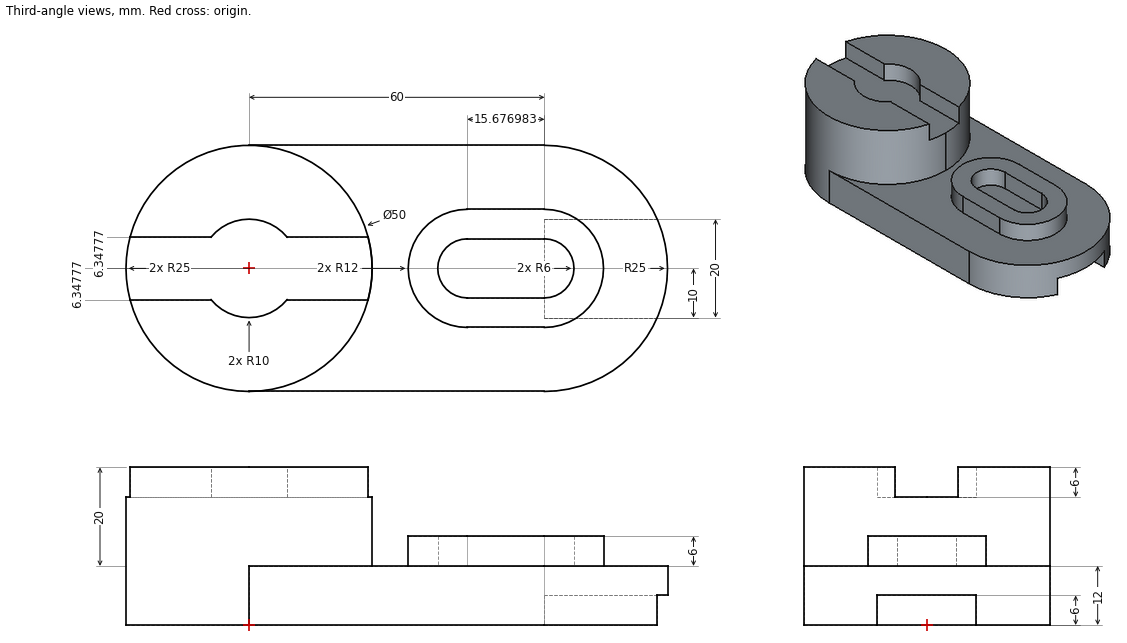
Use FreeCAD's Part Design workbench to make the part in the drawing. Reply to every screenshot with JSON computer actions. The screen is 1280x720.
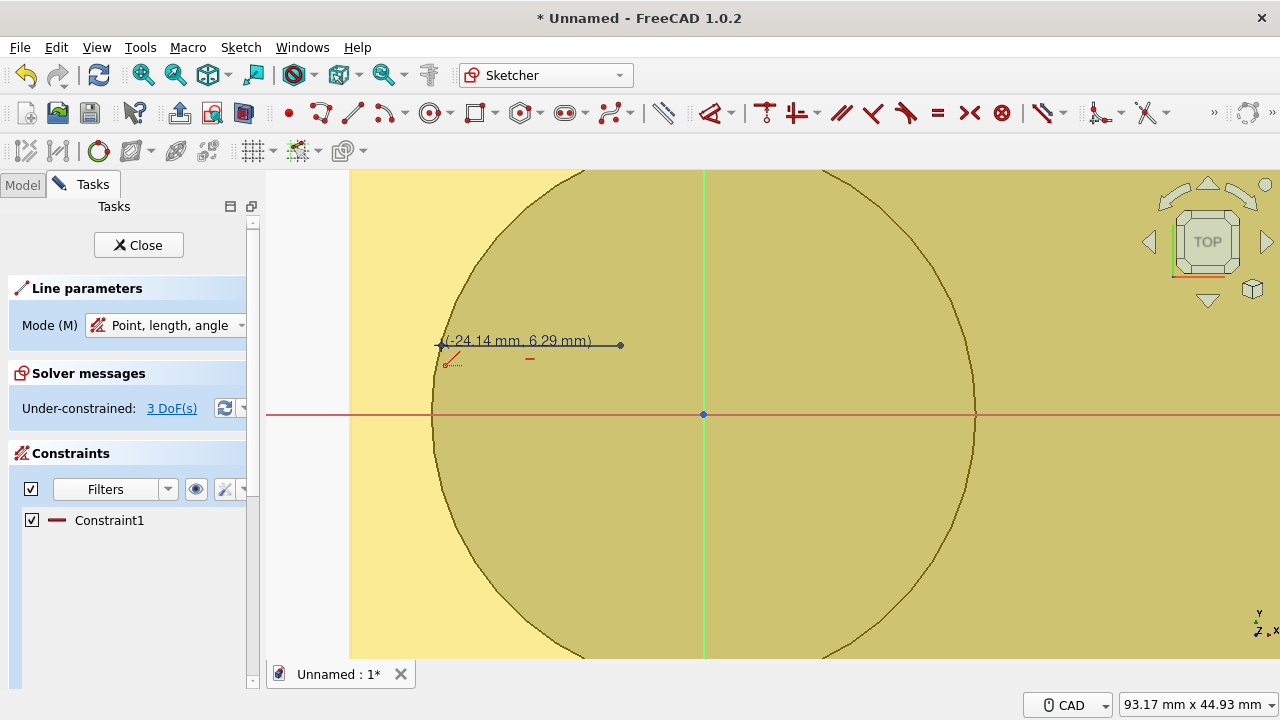
{"action": "left_click", "coordinate": [441, 484]}
{"action": "left_click", "coordinate": [620, 484]}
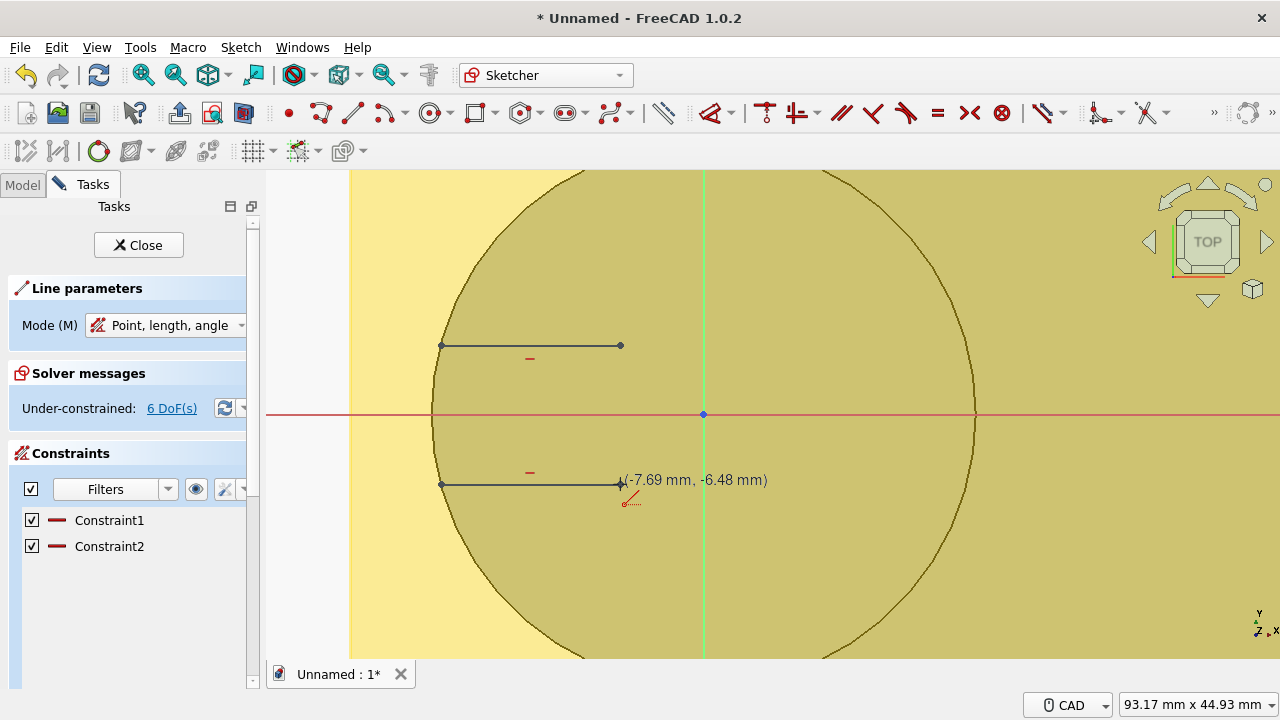
{"action": "left_click", "coordinate": [788, 484]}
{"action": "left_click", "coordinate": [967, 484]}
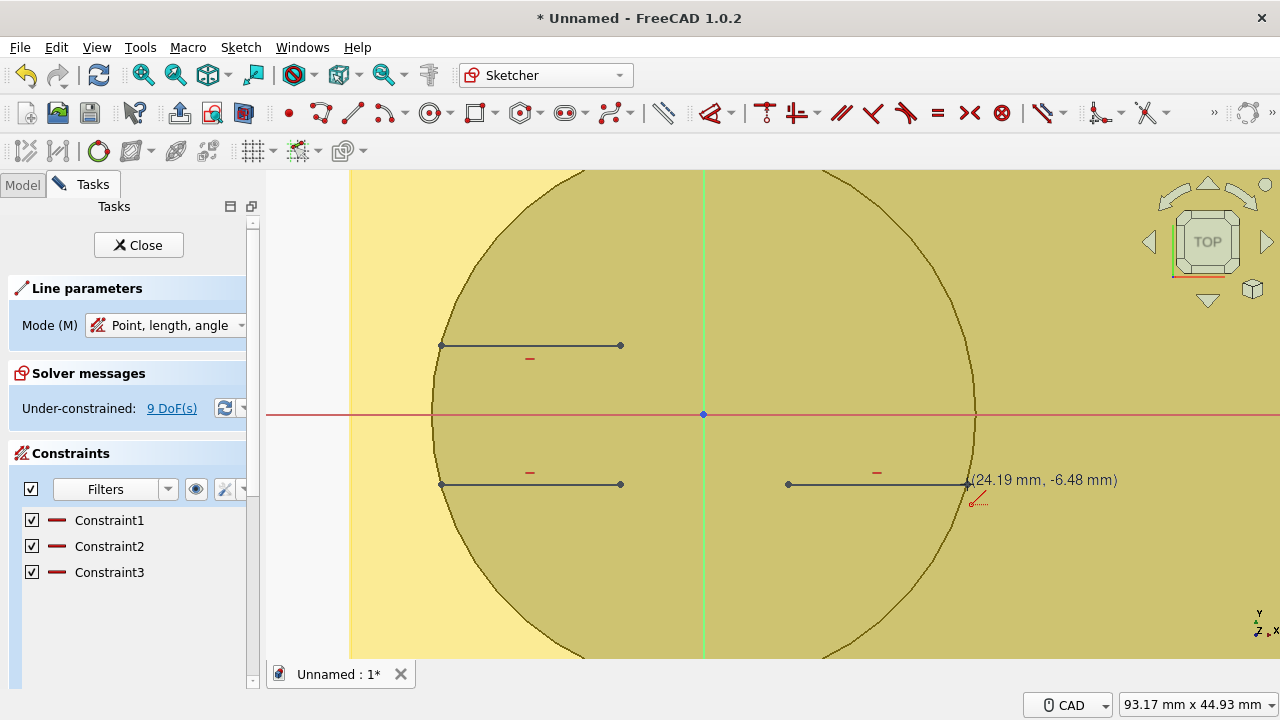
{"action": "left_click", "coordinate": [967, 345]}
{"action": "left_click", "coordinate": [788, 345]}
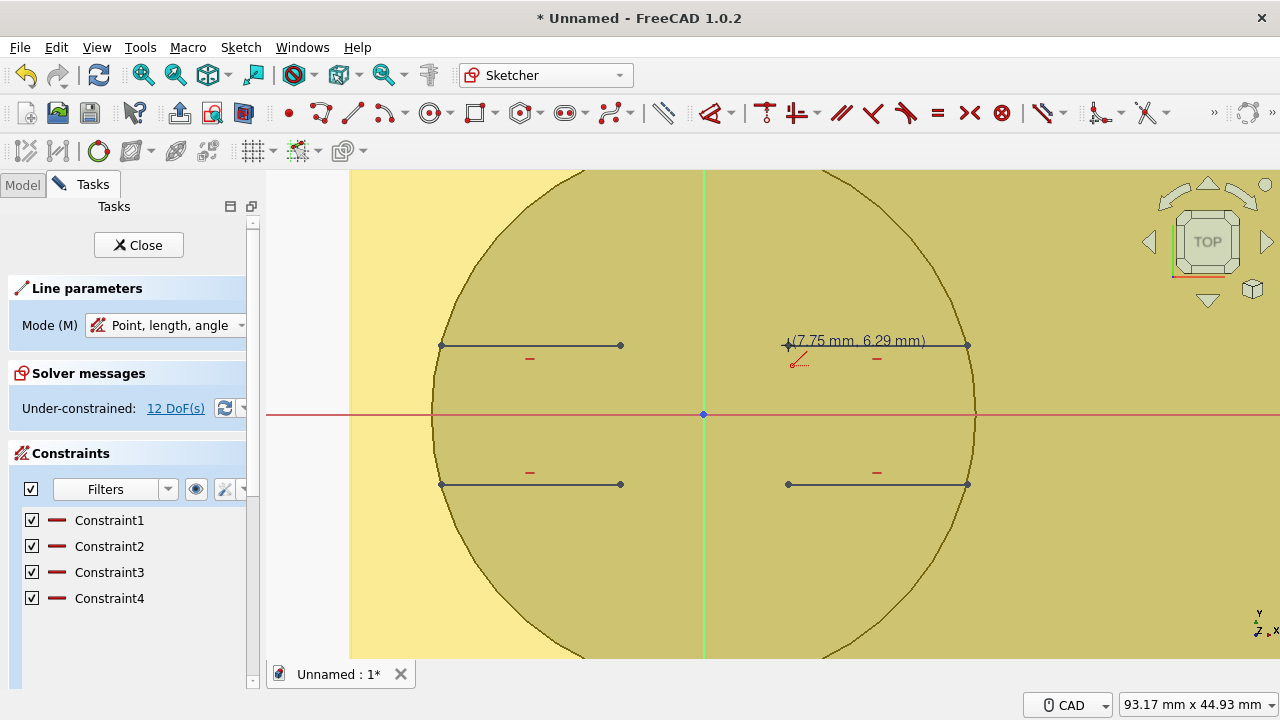
{"action": "key", "text": "g 3 a"}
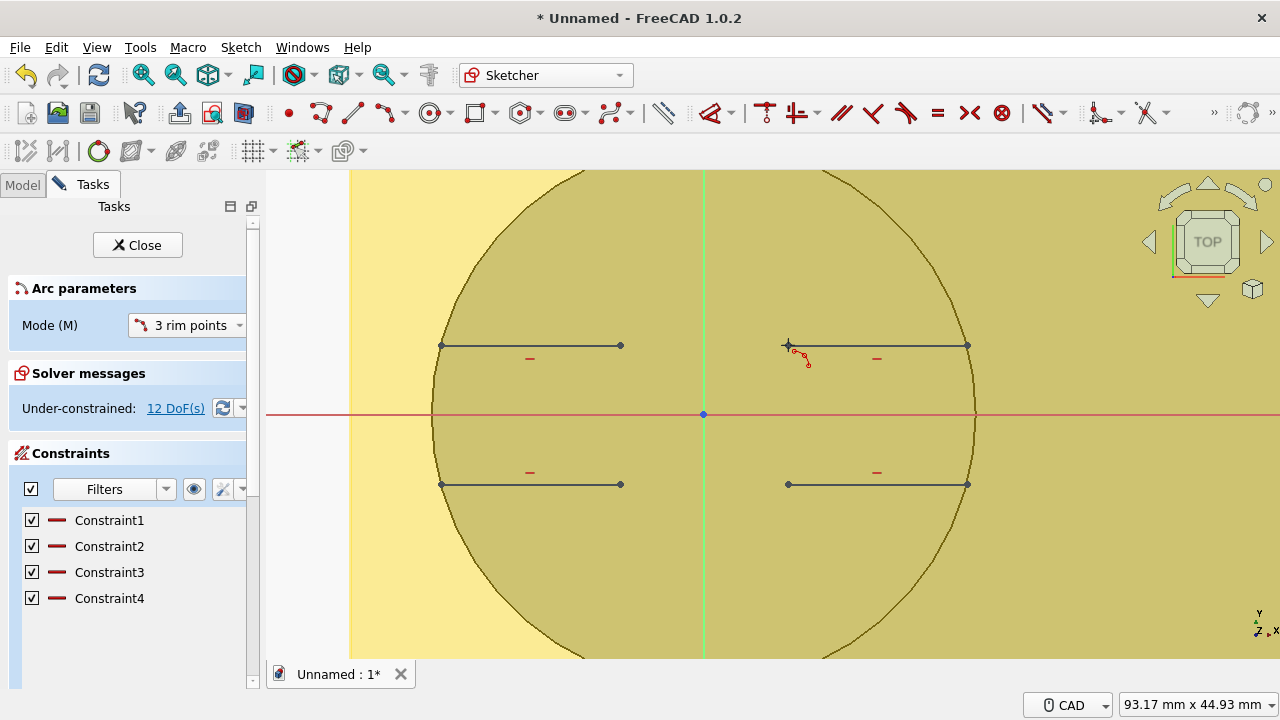
{"action": "left_click", "coordinate": [441, 346]}
{"action": "left_click", "coordinate": [441, 485]}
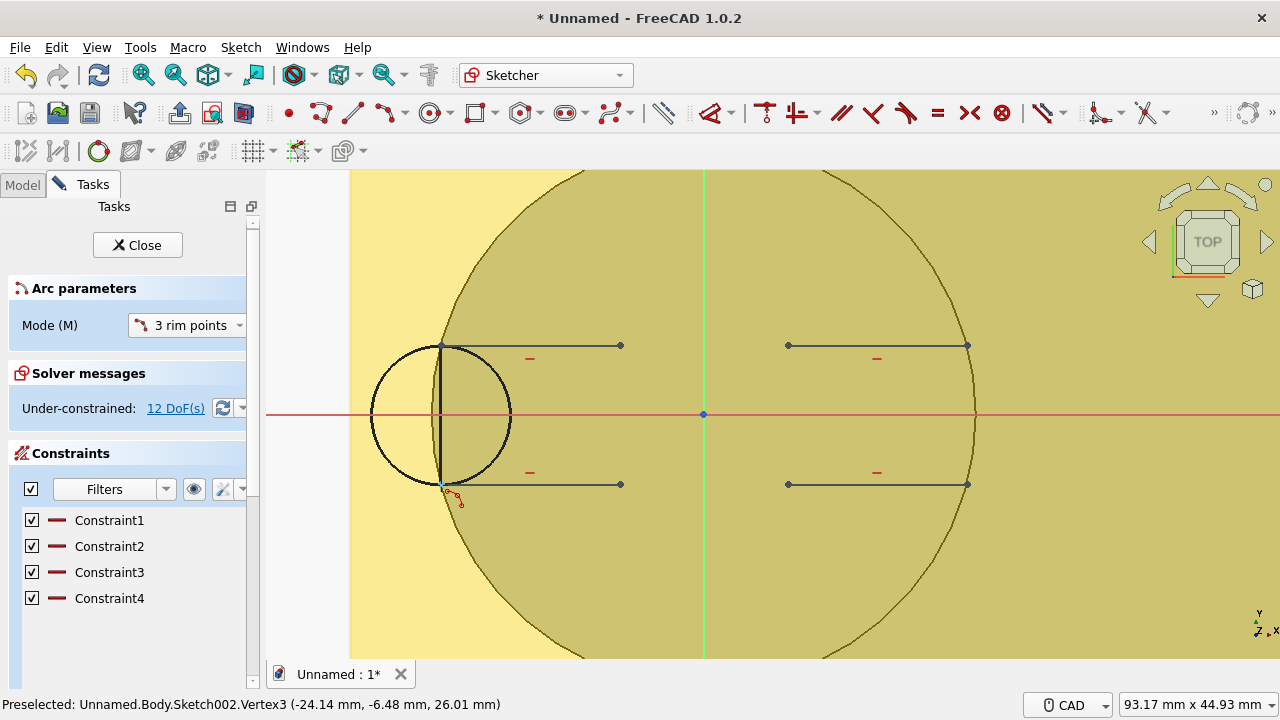
{"action": "scroll", "coordinate": [432, 401], "scroll_direction": "up", "scroll_amount": 4}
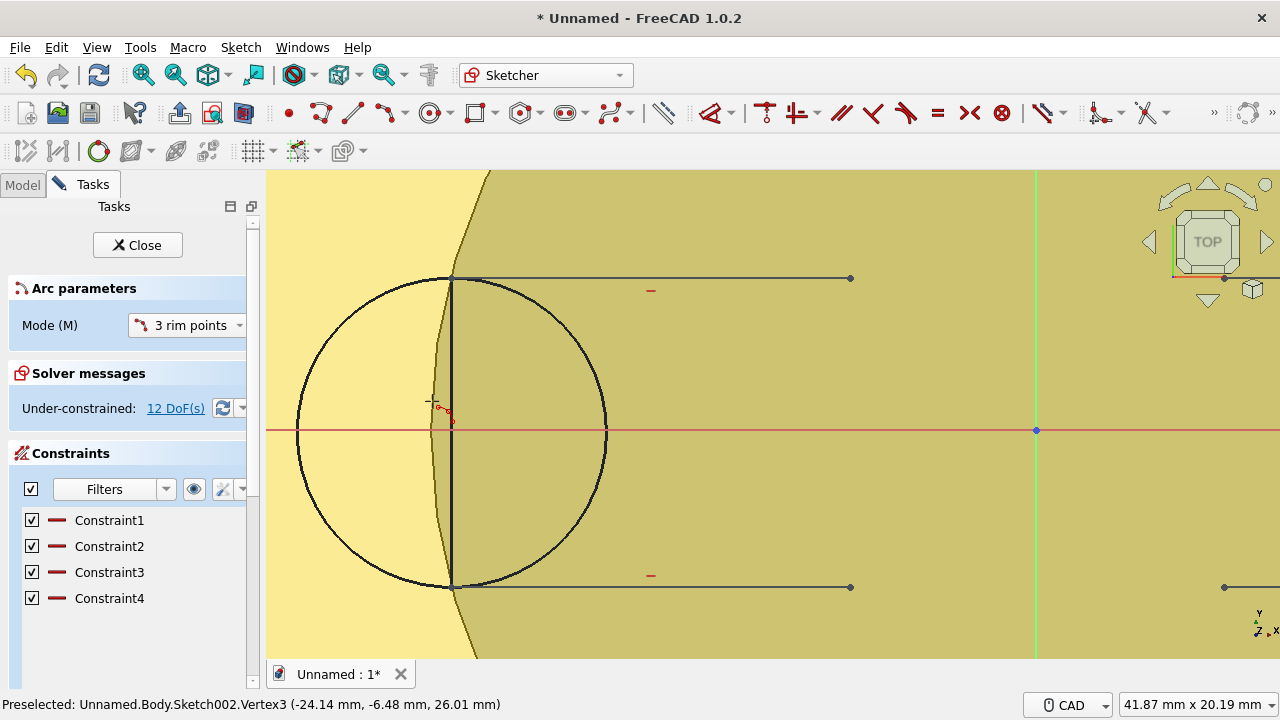
{"action": "left_click", "coordinate": [432, 399]}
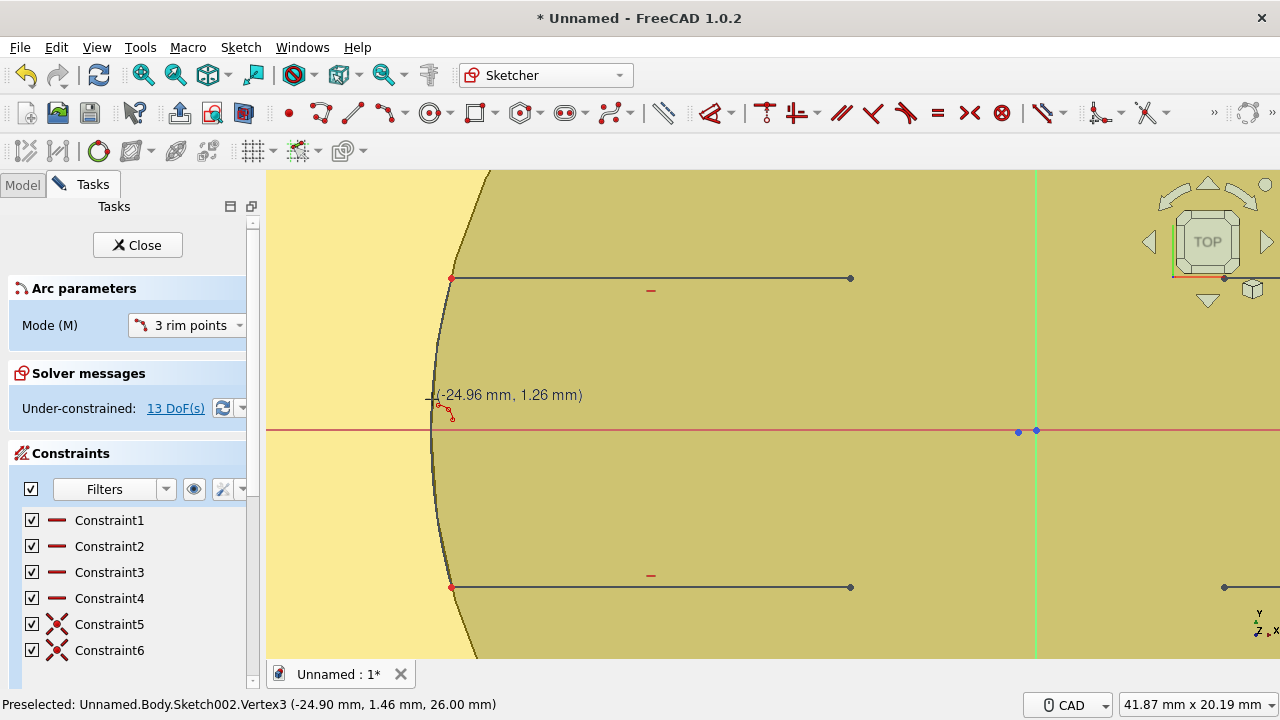
{"action": "left_click", "coordinate": [850, 587]}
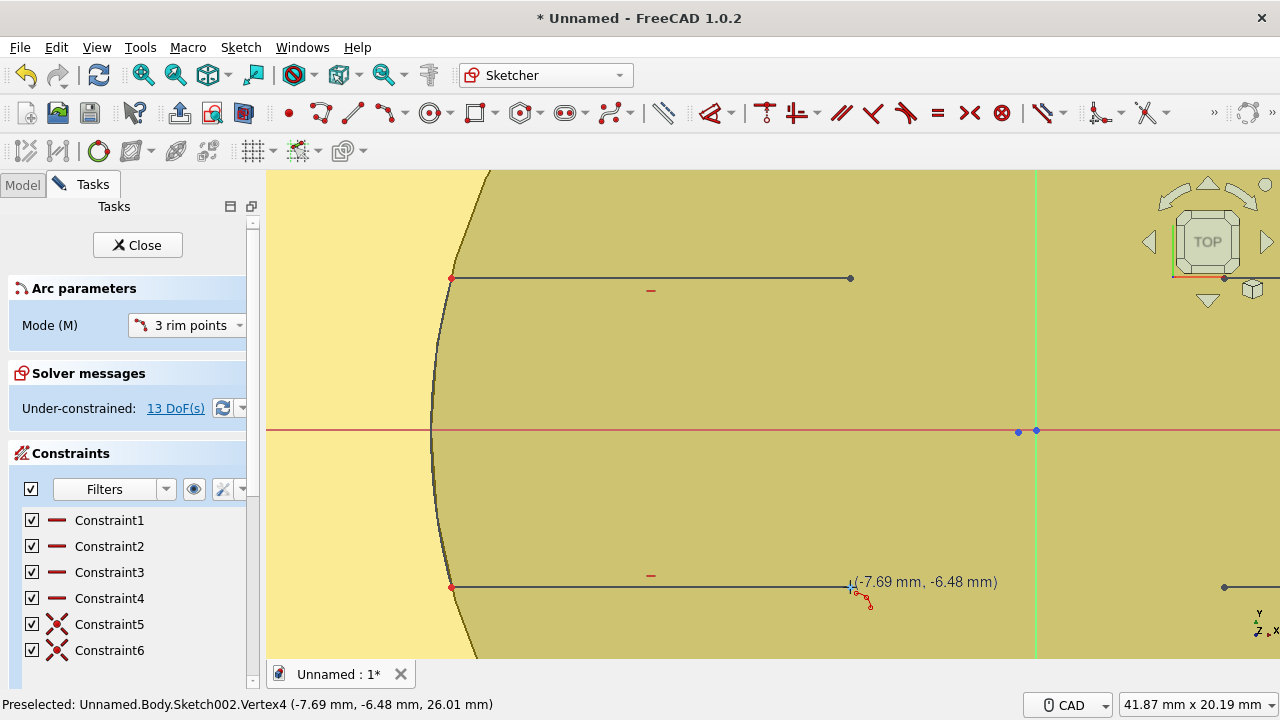
{"action": "scroll", "coordinate": [434, 401], "scroll_direction": "down", "scroll_amount": 4}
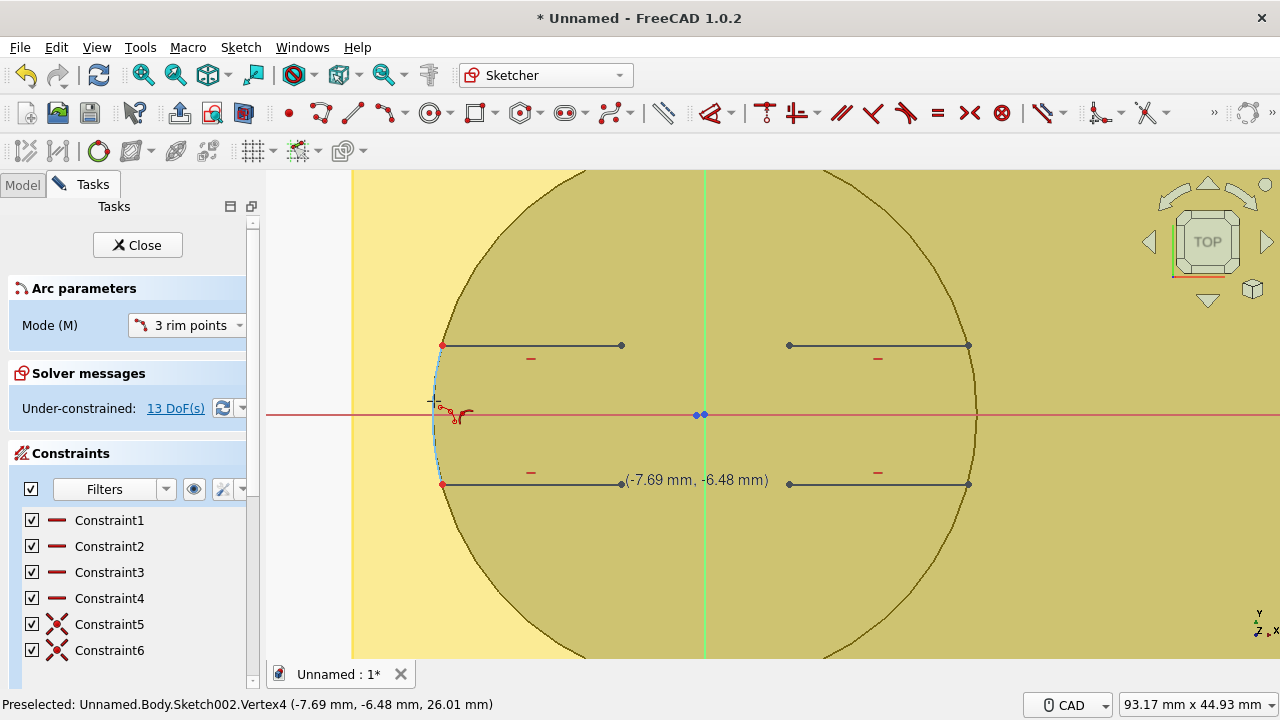
{"action": "left_click", "coordinate": [789, 485]}
{"action": "left_click", "coordinate": [686, 522]}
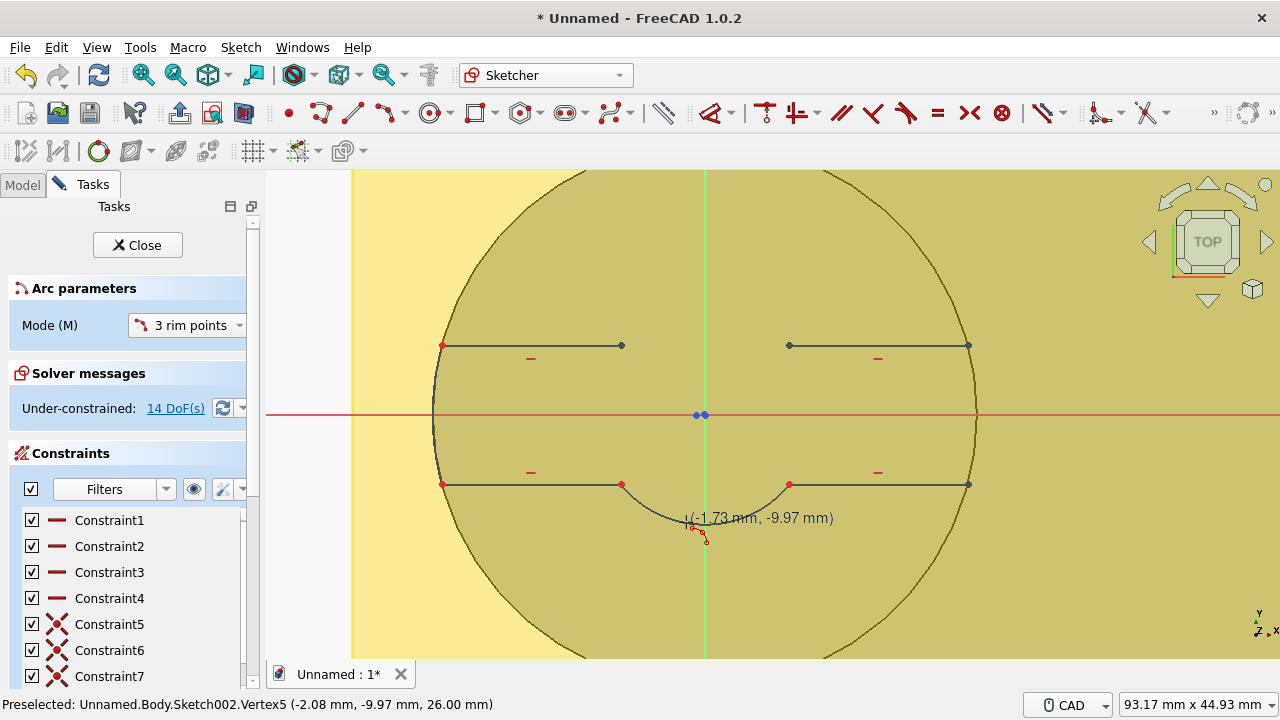
{"action": "left_click", "coordinate": [968, 485]}
{"action": "left_click", "coordinate": [968, 346]}